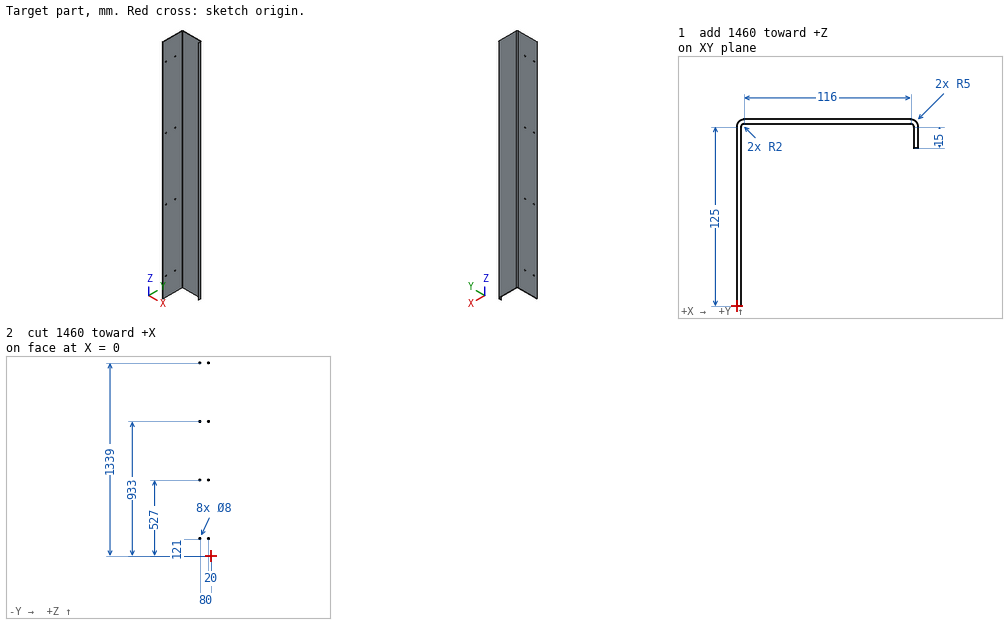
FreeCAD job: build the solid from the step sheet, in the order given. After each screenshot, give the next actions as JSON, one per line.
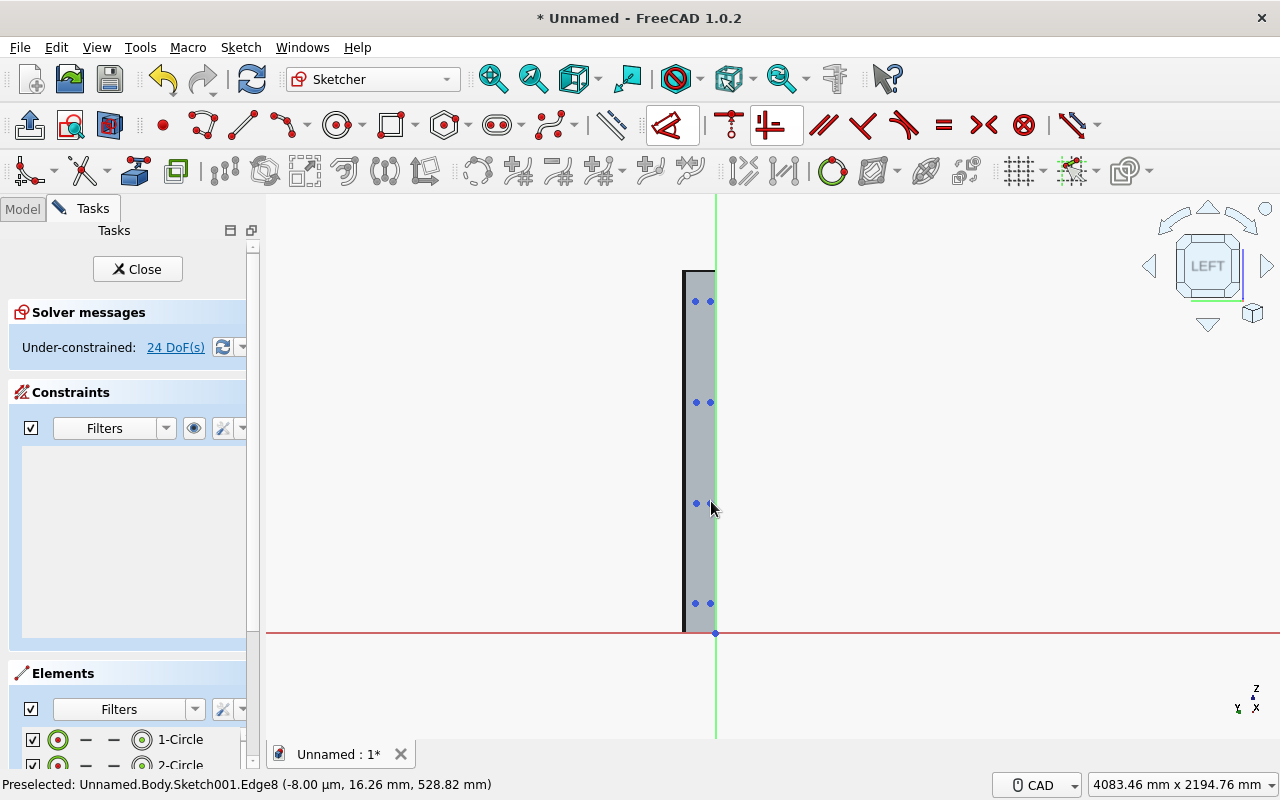
{"action": "scroll", "coordinate": [697, 603], "scroll_direction": "up", "scroll_amount": 12}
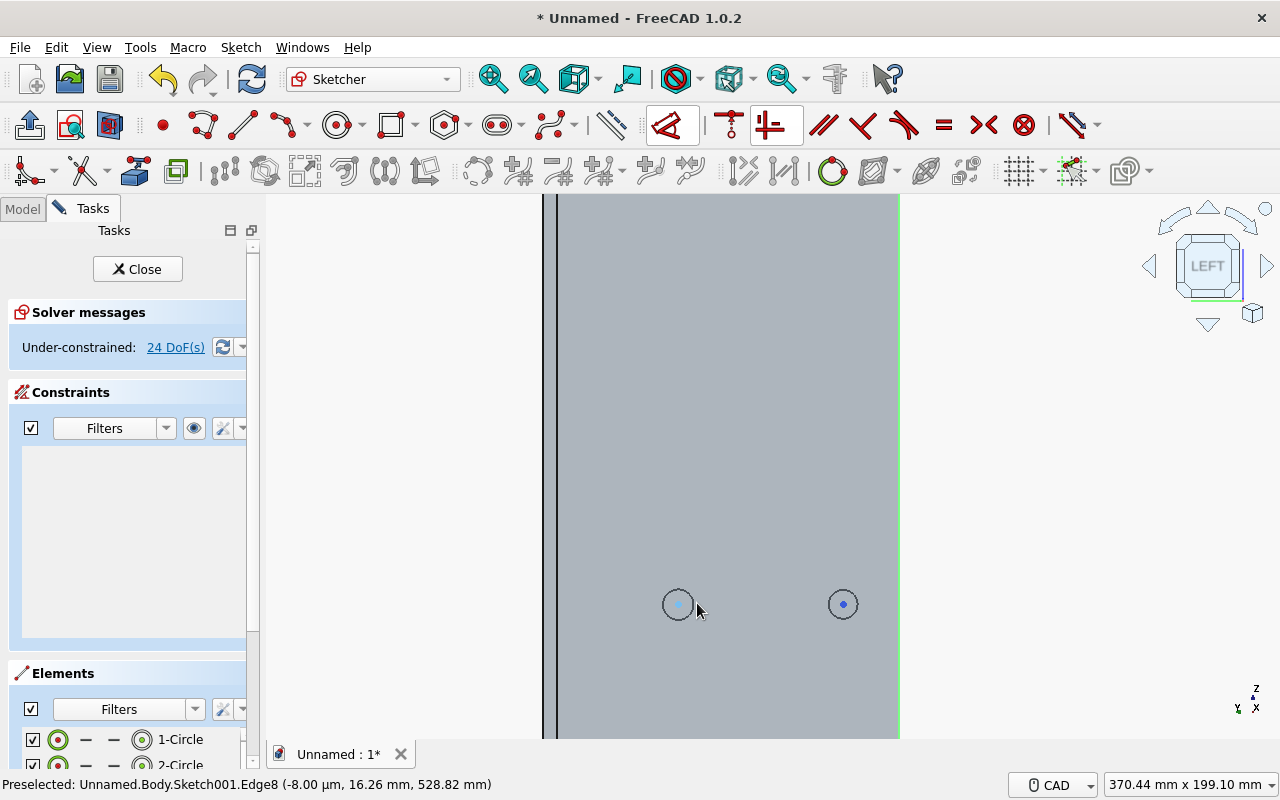
{"action": "left_click", "coordinate": [689, 594]}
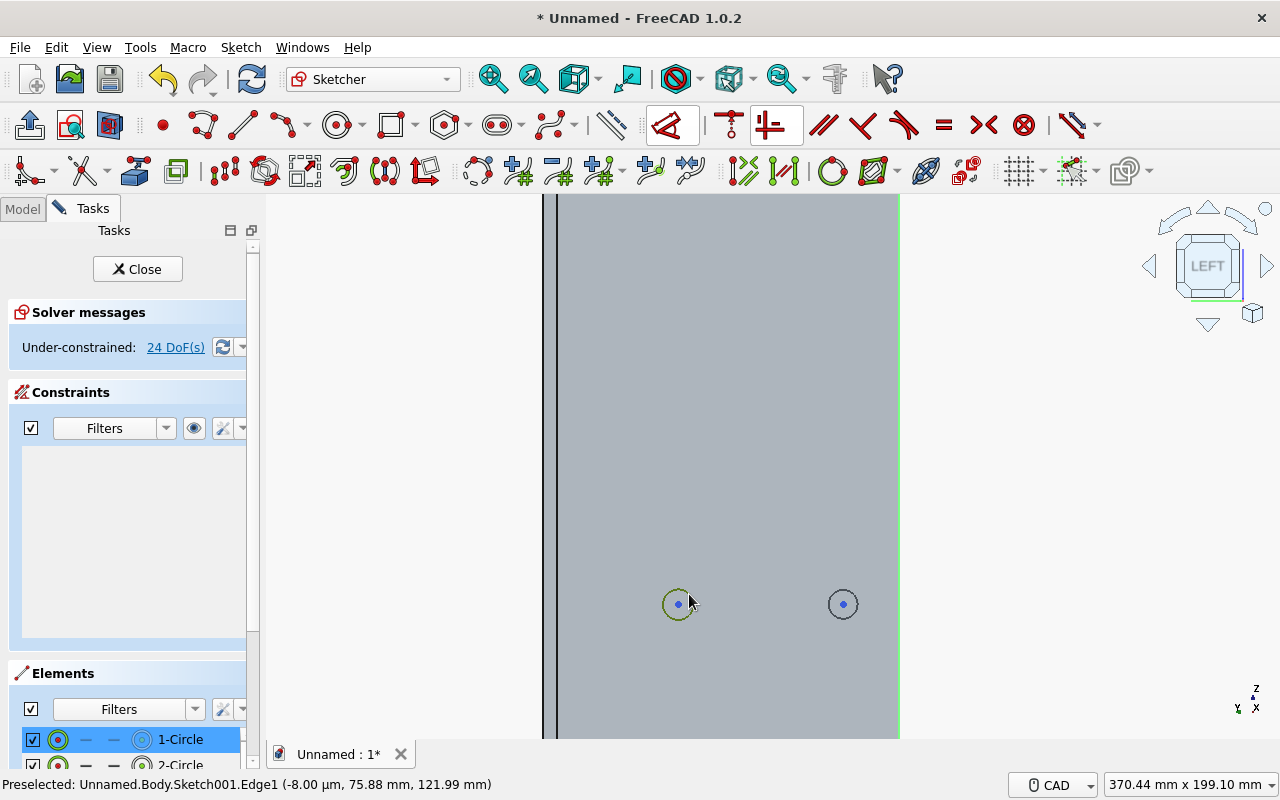
{"action": "scroll", "coordinate": [697, 604], "scroll_direction": "down", "scroll_amount": 12}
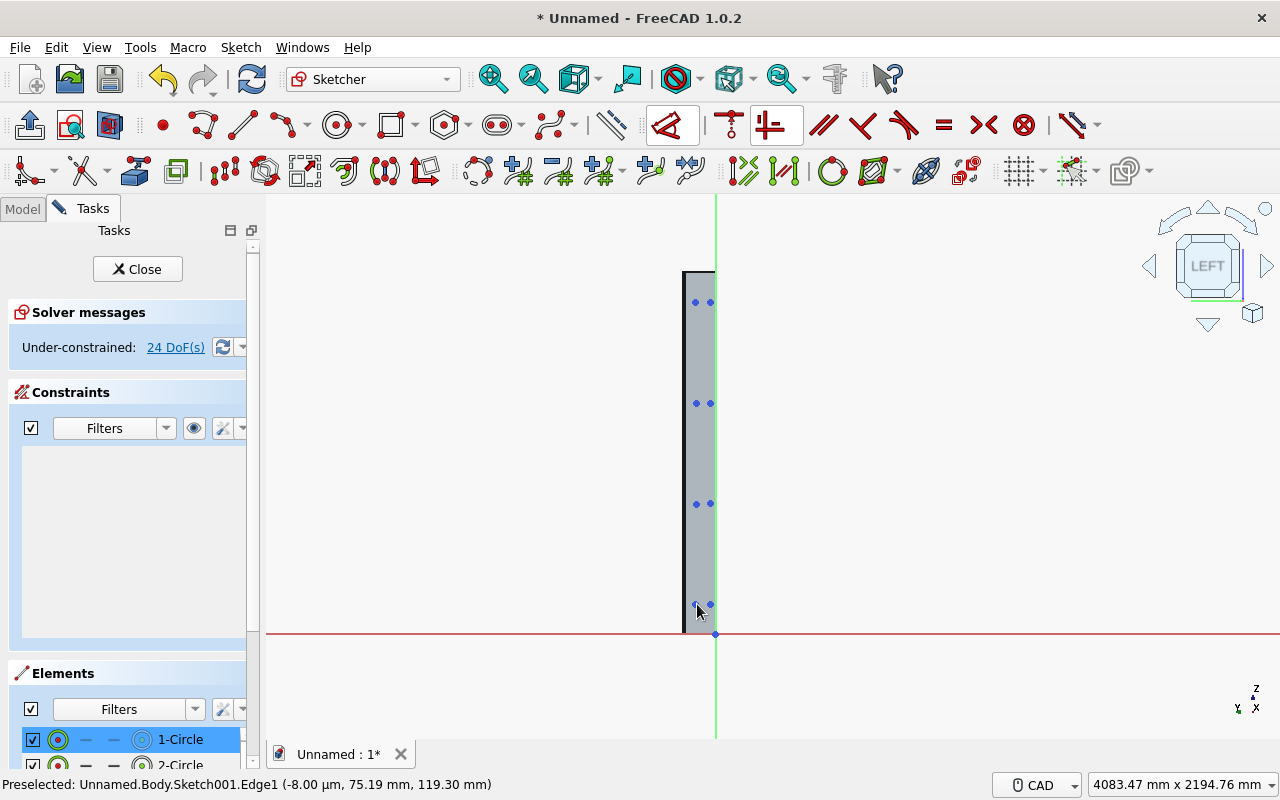
{"action": "scroll", "coordinate": [697, 301], "scroll_direction": "up", "scroll_amount": 11}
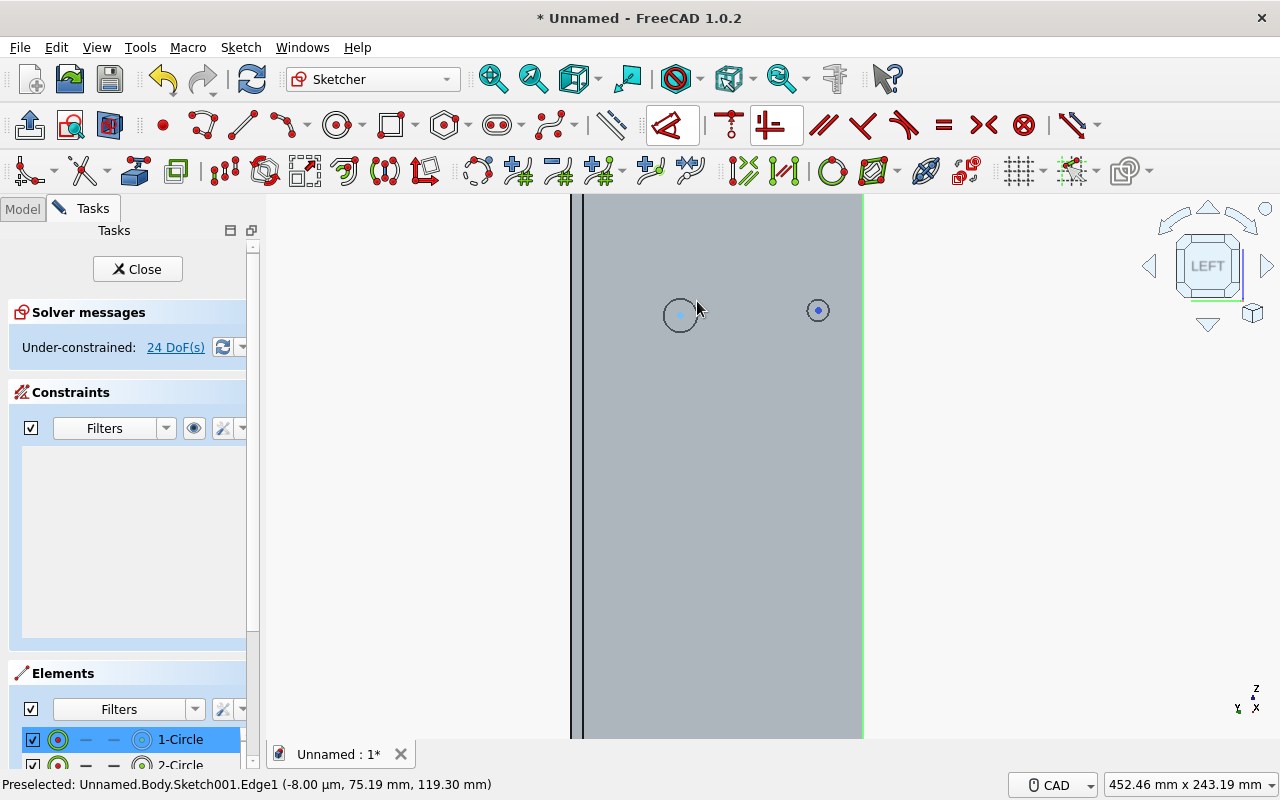
{"action": "left_click", "coordinate": [692, 304]}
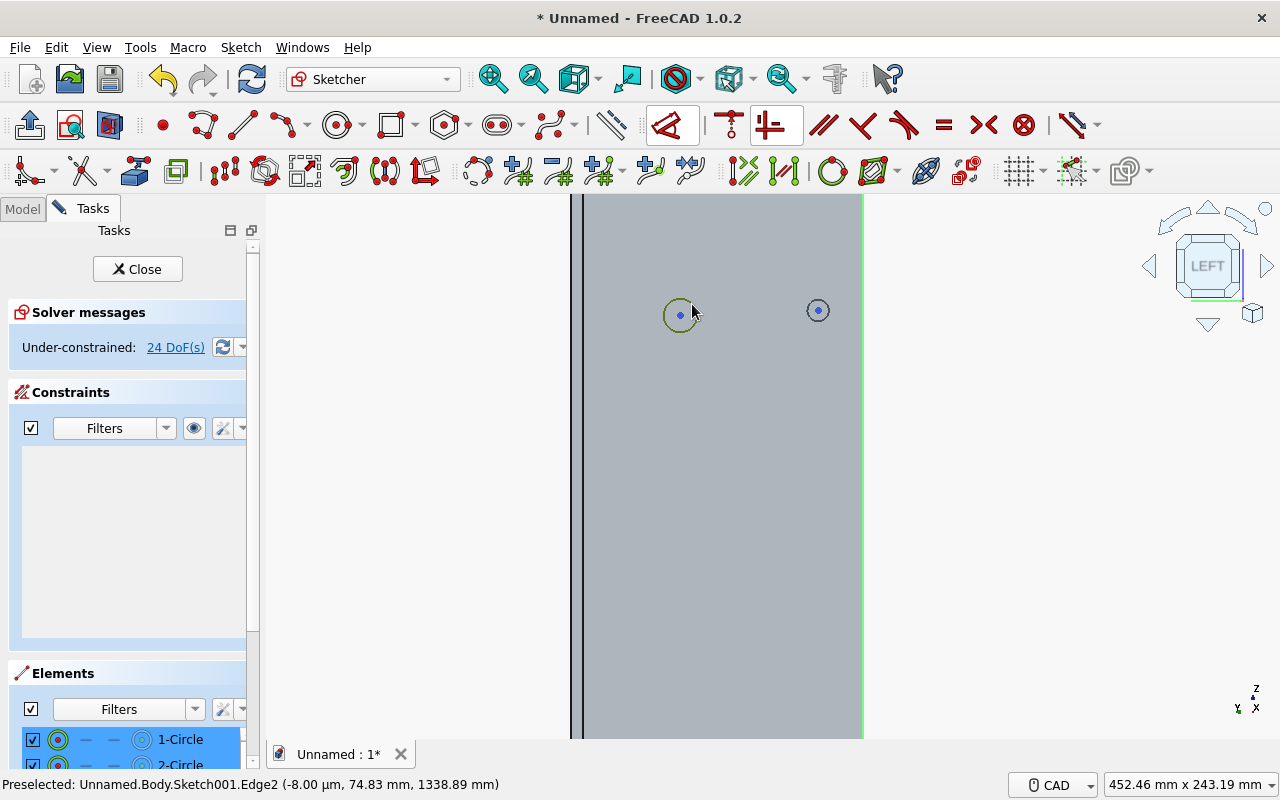
{"action": "scroll", "coordinate": [697, 300], "scroll_direction": "down", "scroll_amount": 11}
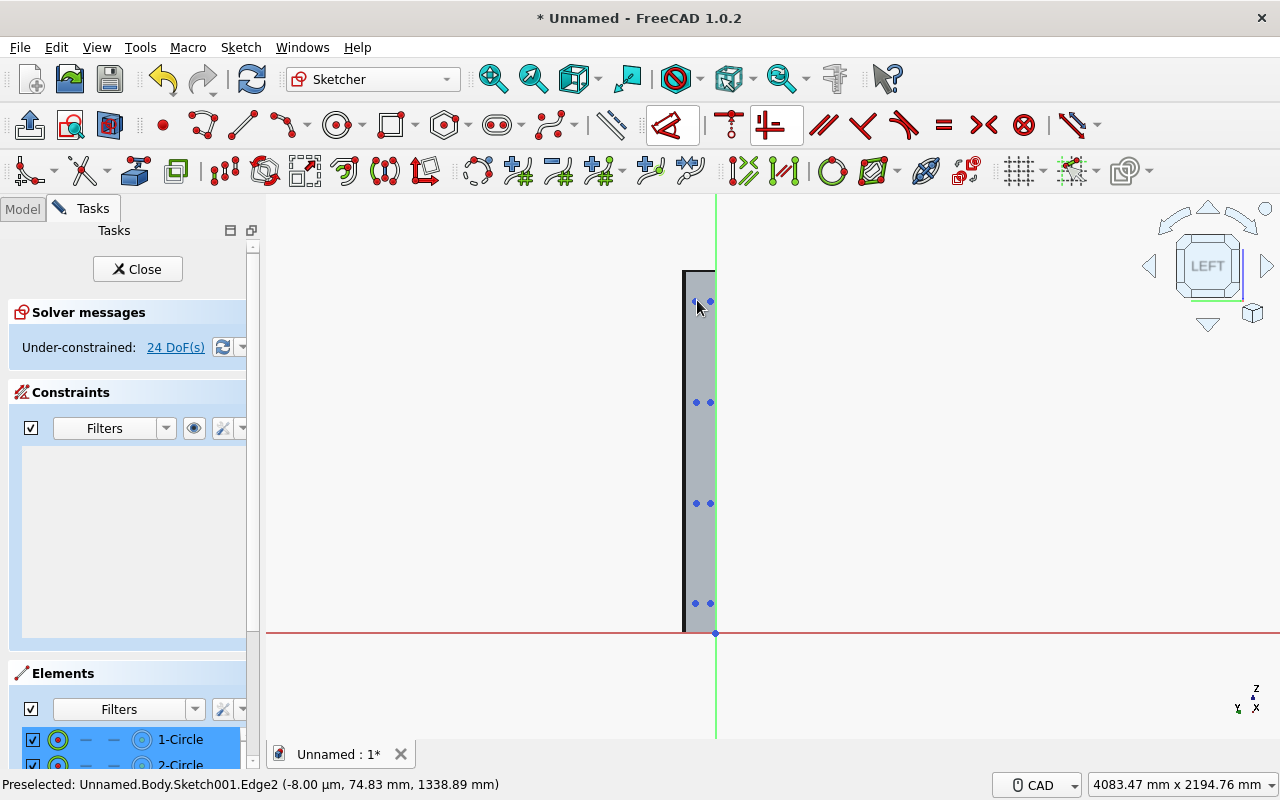
{"action": "scroll", "coordinate": [697, 402], "scroll_direction": "up", "scroll_amount": 11}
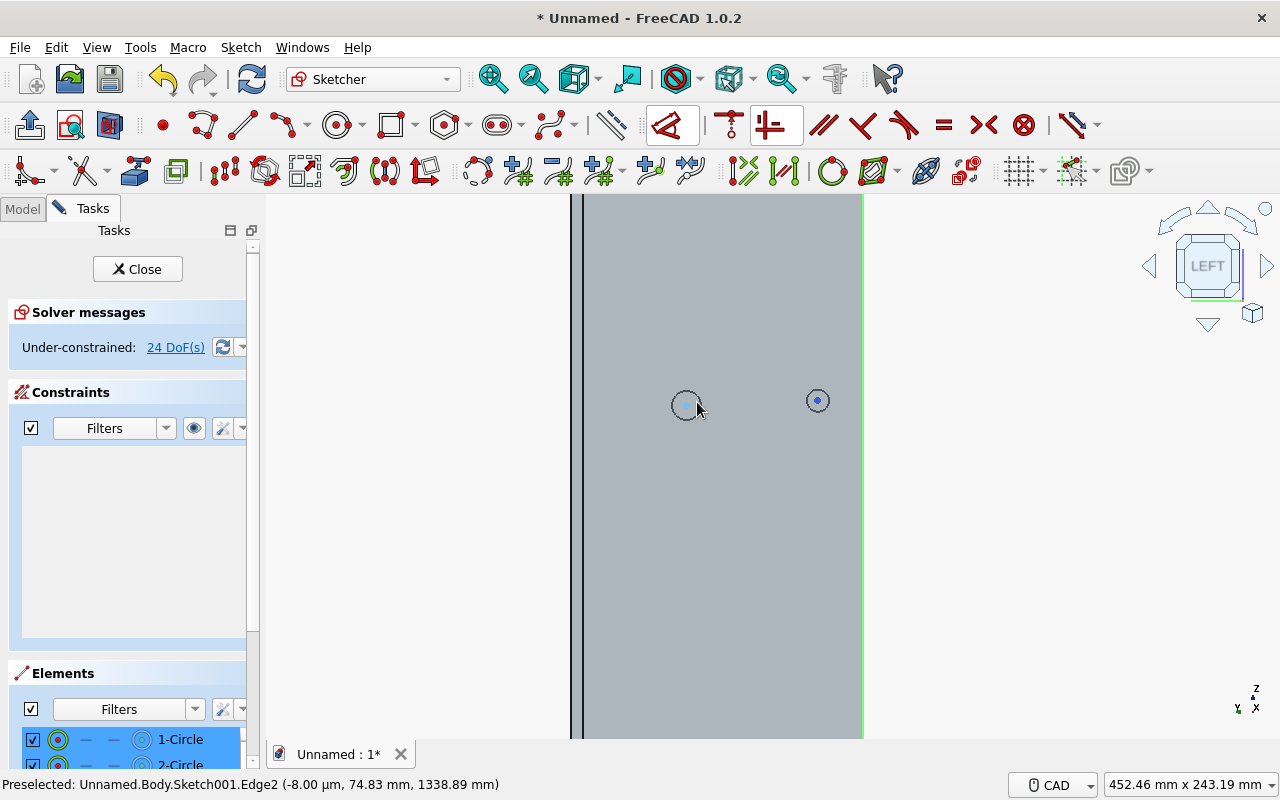
{"action": "left_click", "coordinate": [697, 395]}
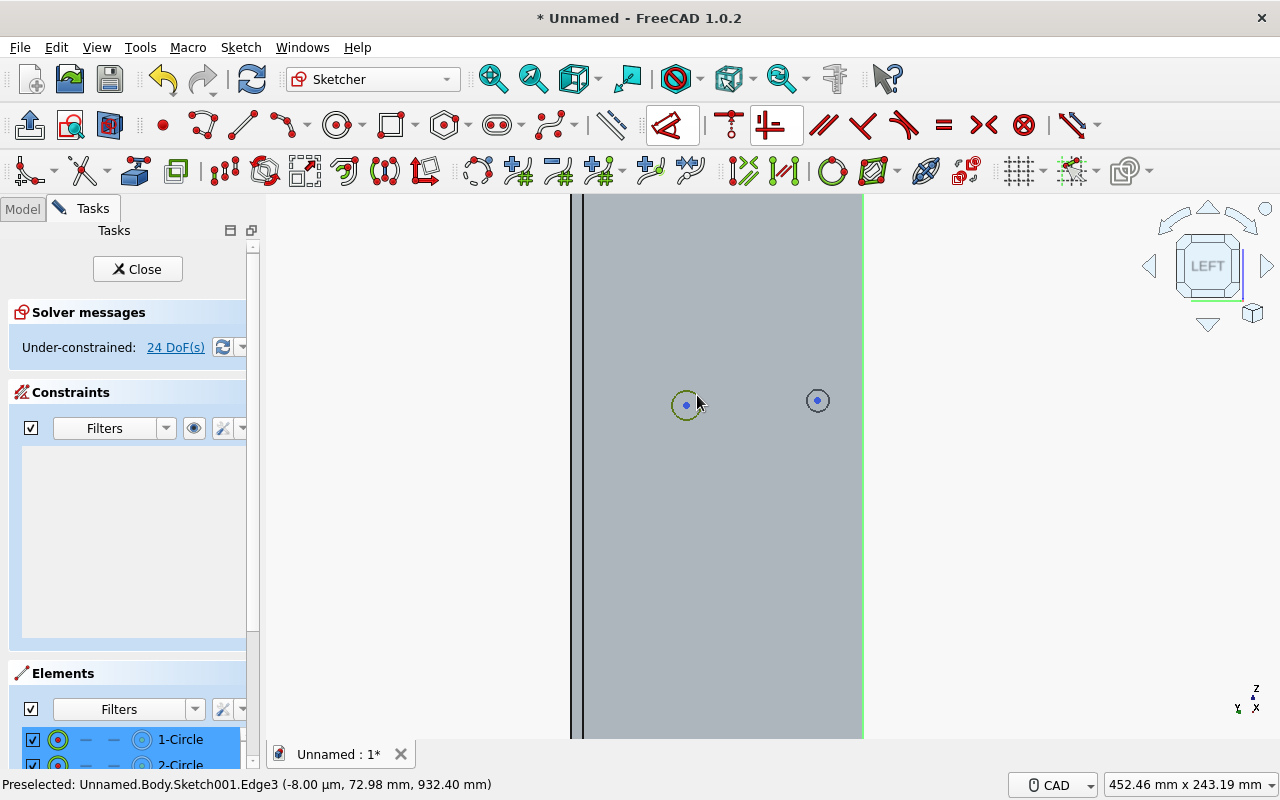
{"action": "scroll", "coordinate": [697, 402], "scroll_direction": "down", "scroll_amount": 11}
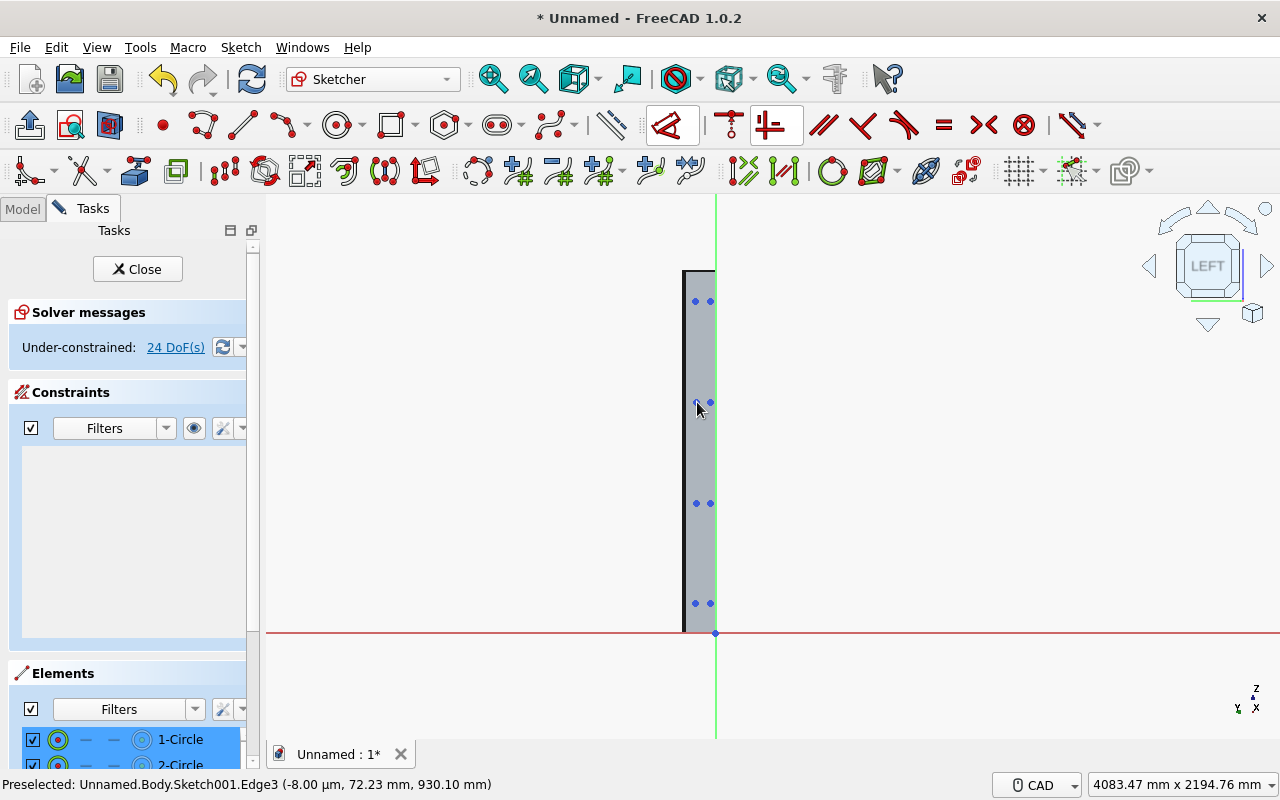
{"action": "scroll", "coordinate": [697, 502], "scroll_direction": "up", "scroll_amount": 12}